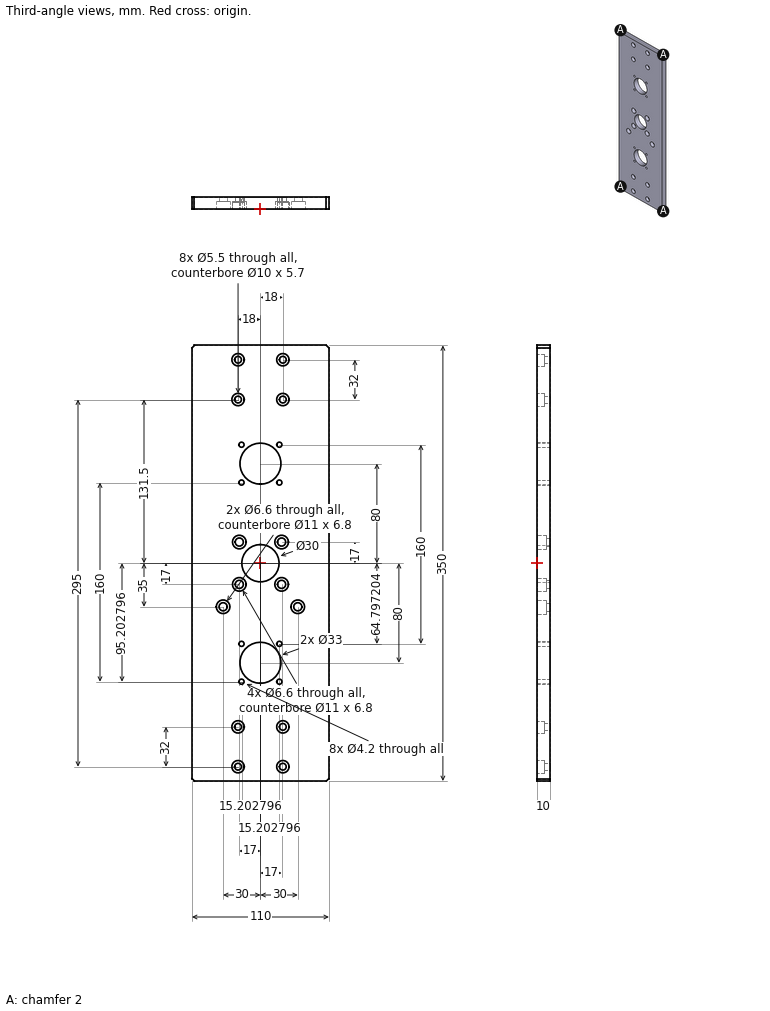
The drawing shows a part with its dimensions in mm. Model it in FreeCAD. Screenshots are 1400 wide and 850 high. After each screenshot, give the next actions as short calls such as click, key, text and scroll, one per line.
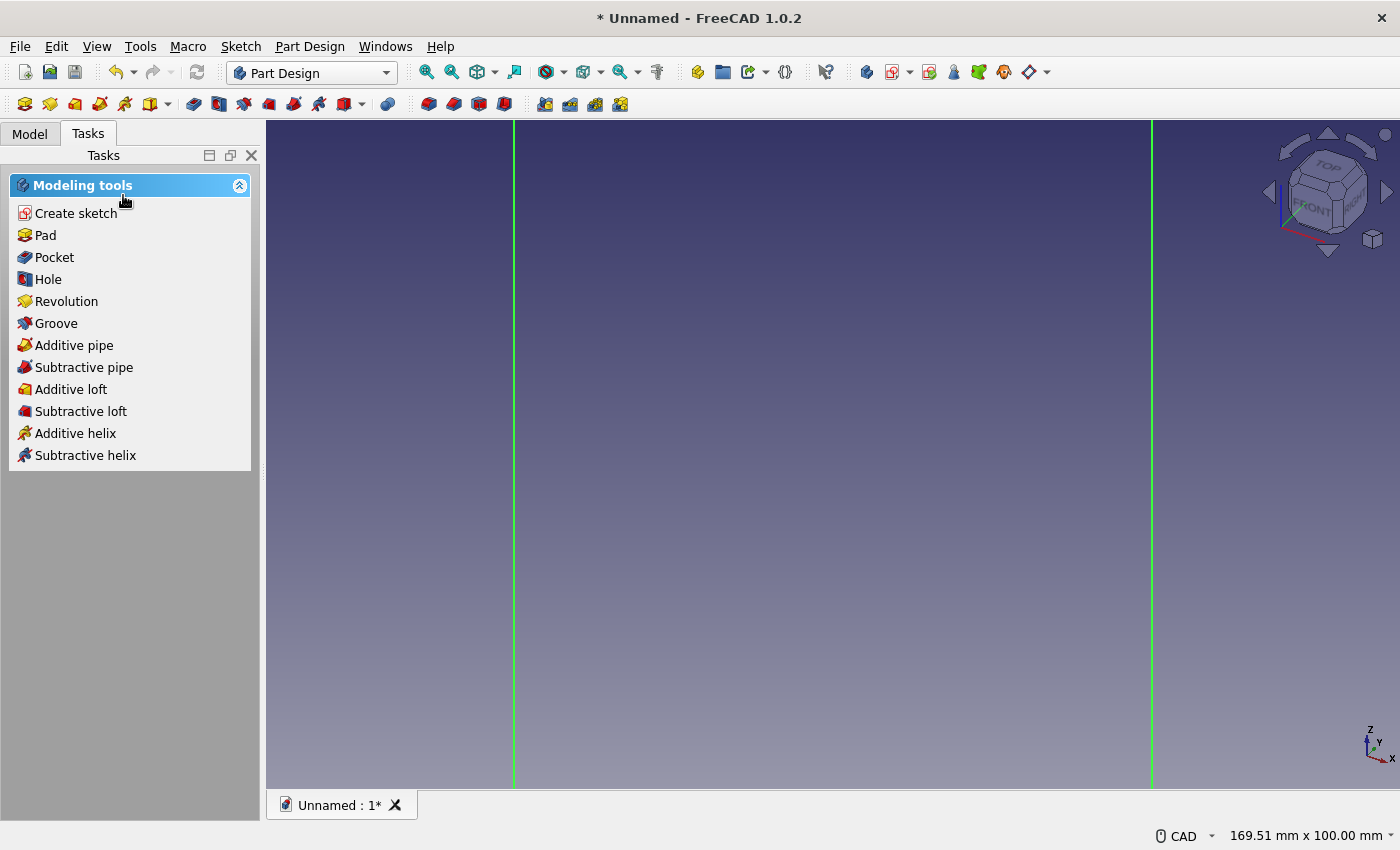
click(25, 104)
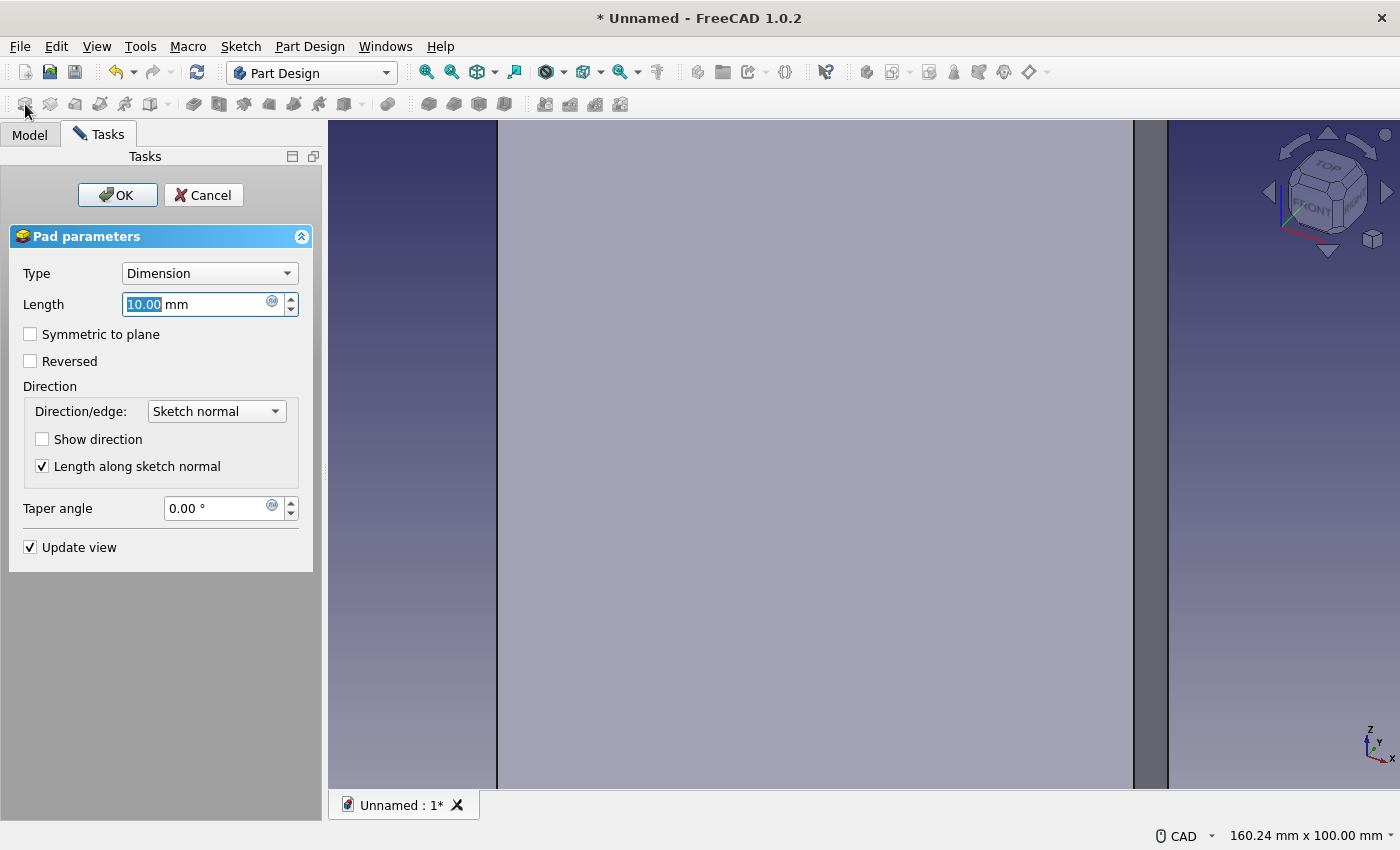
text(10)
key(Tab)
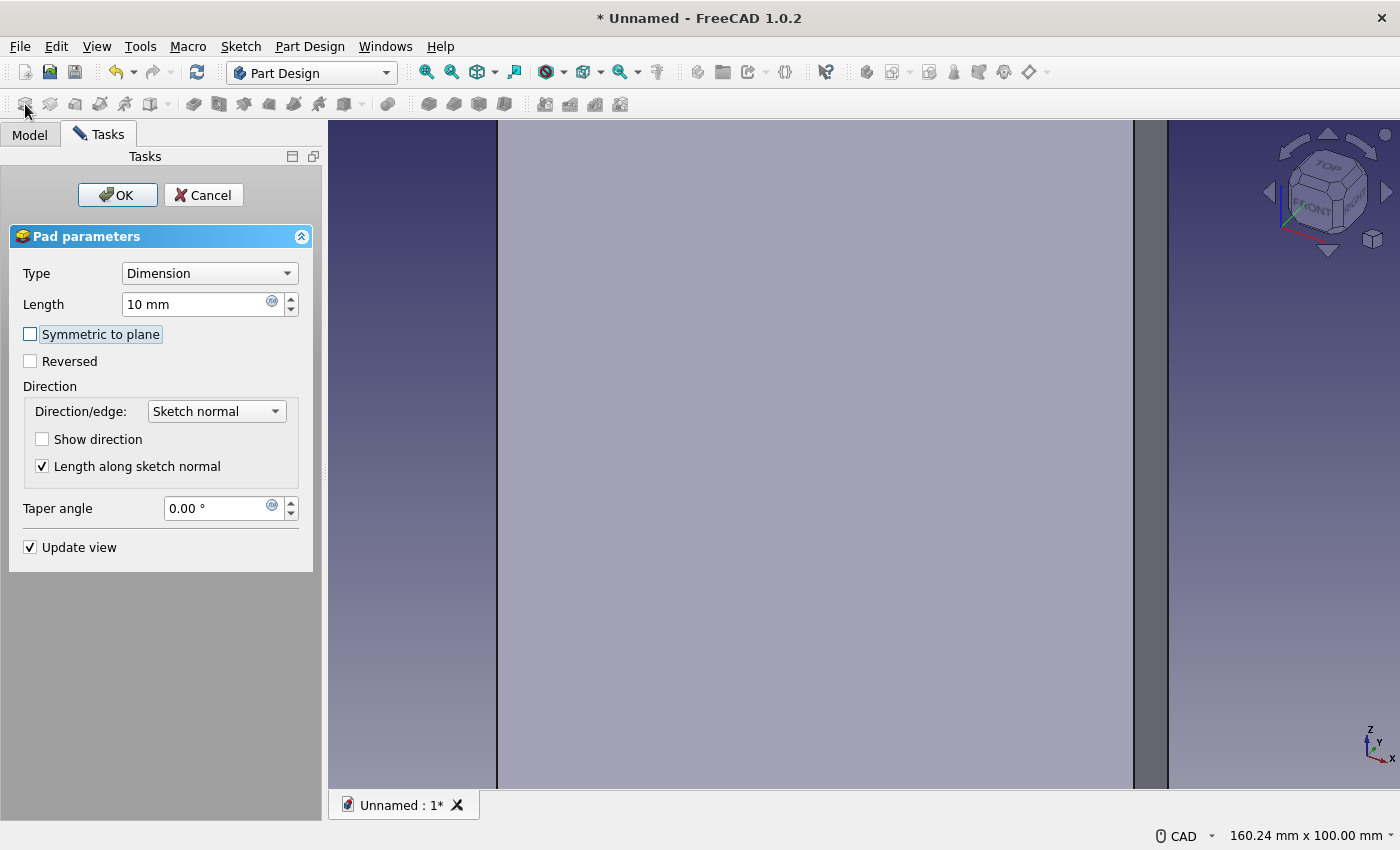
click(31, 361)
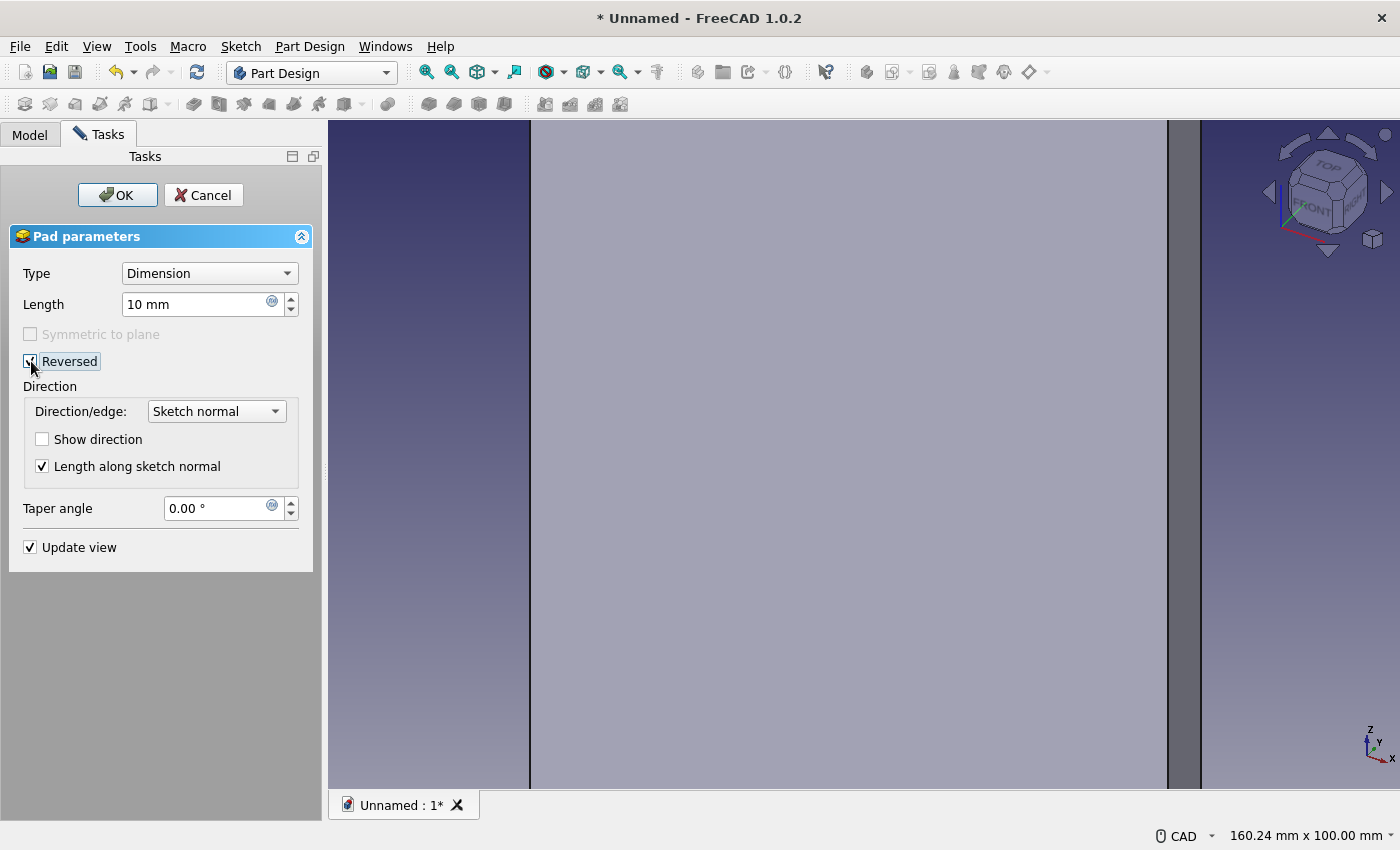
click(118, 195)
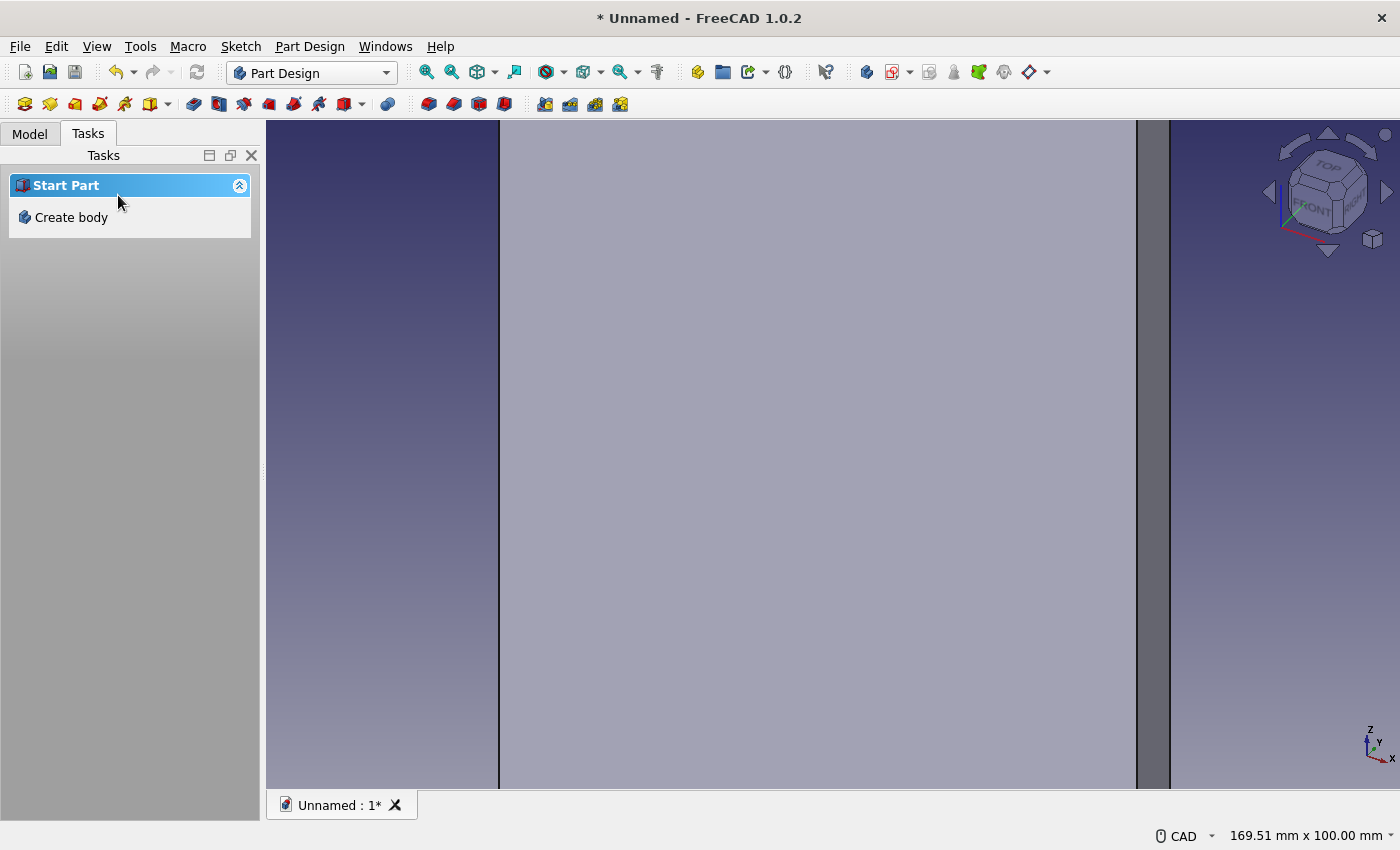
key(v)
key(f)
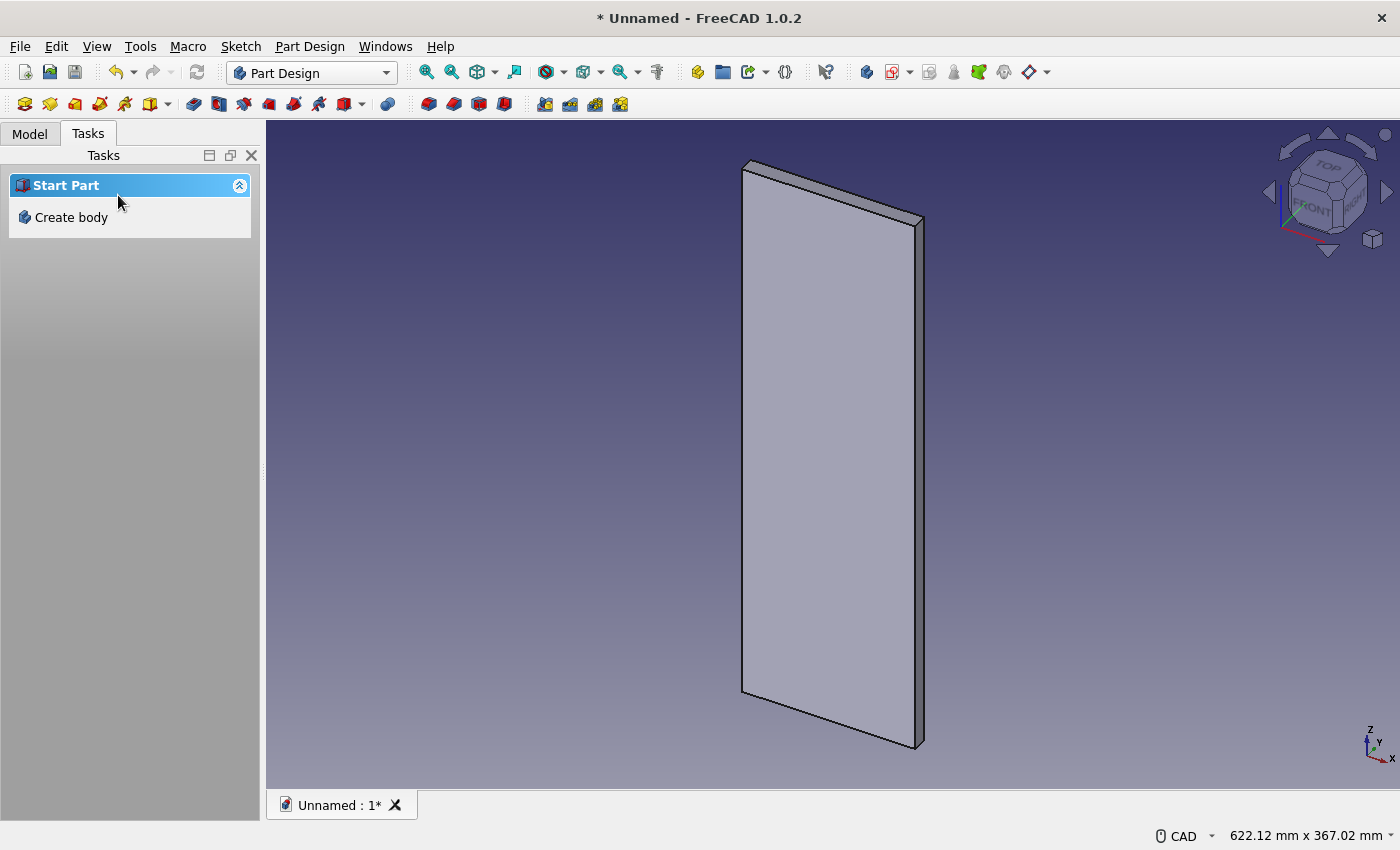
click(892, 72)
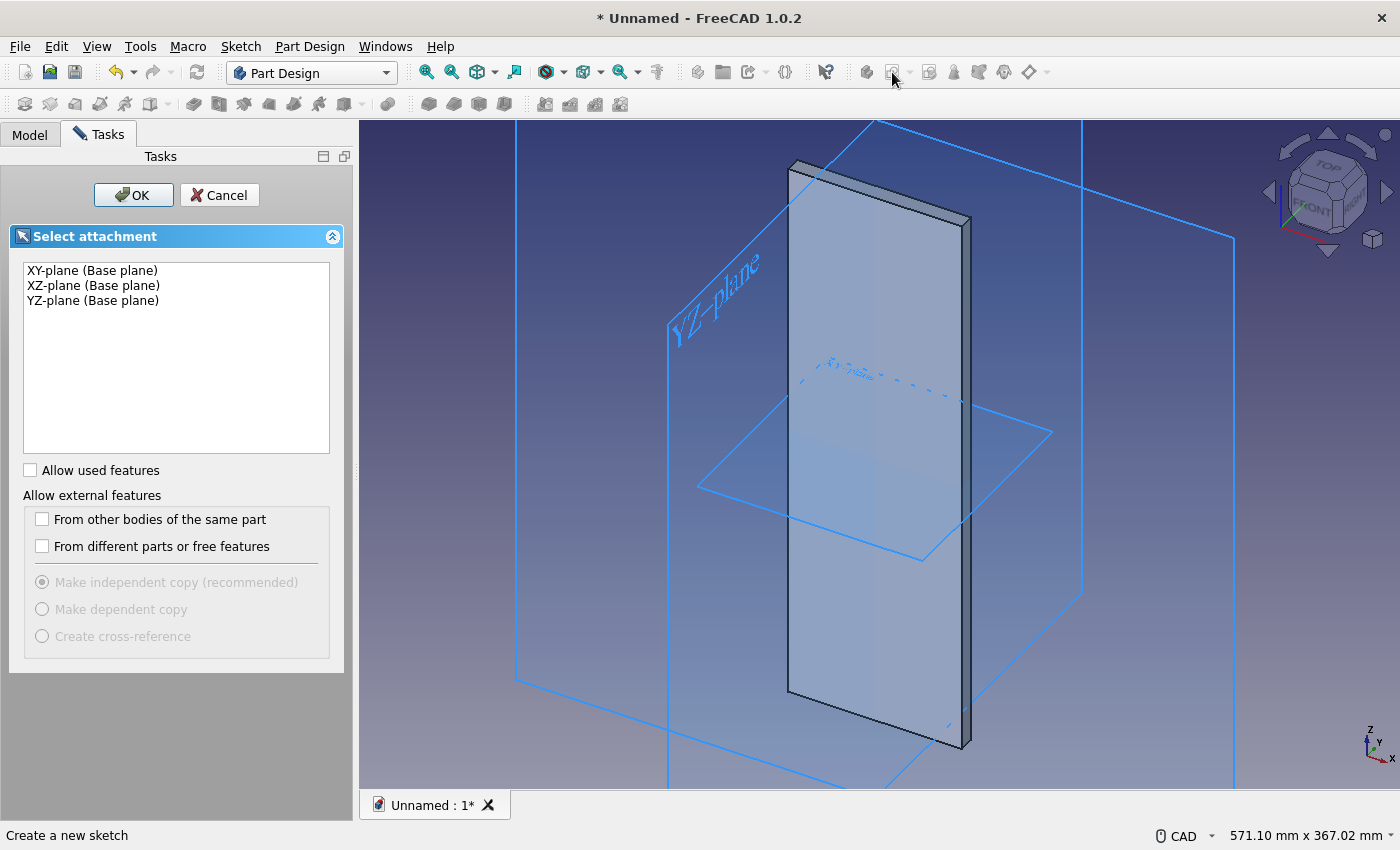
click(84, 286)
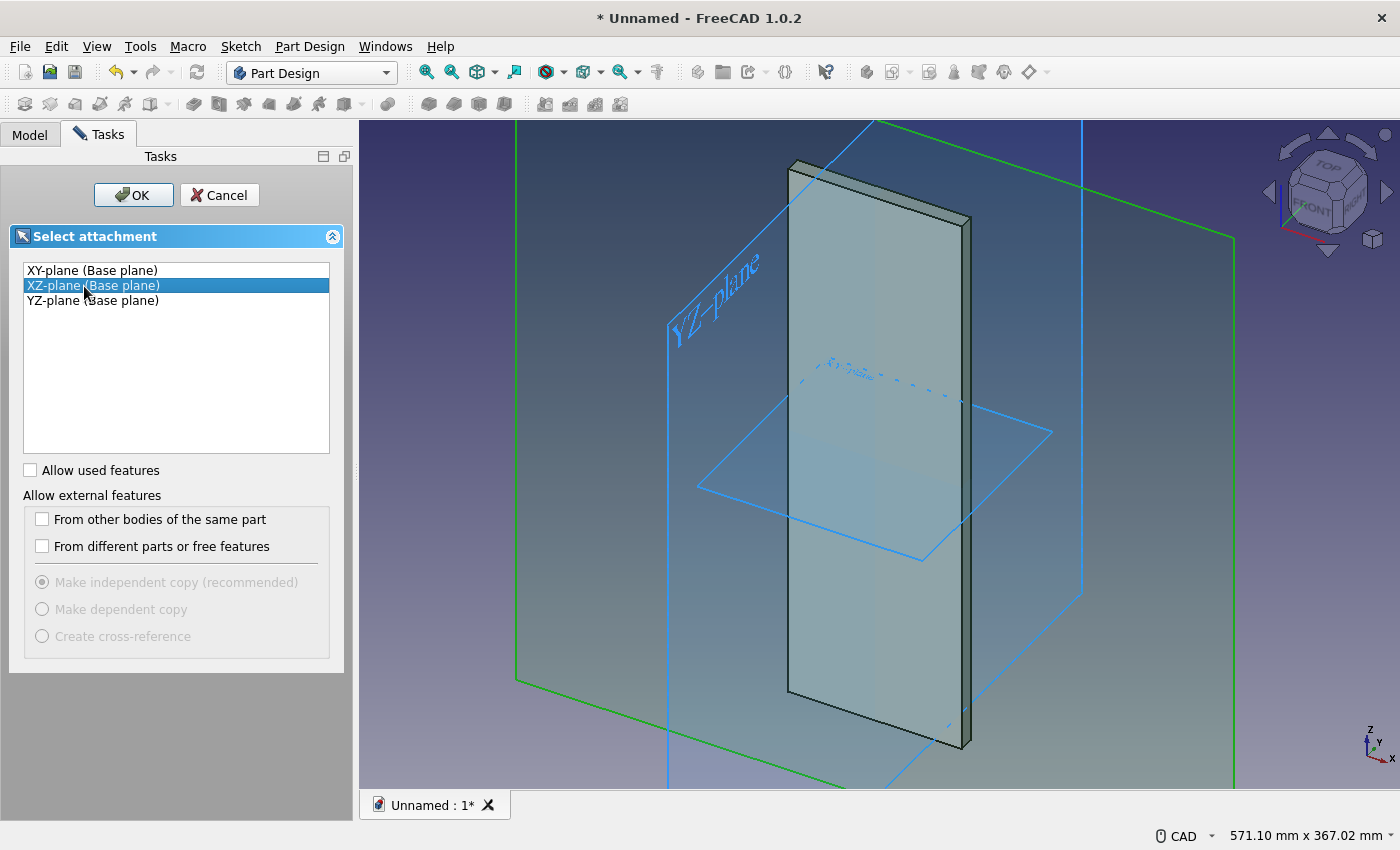
click(134, 195)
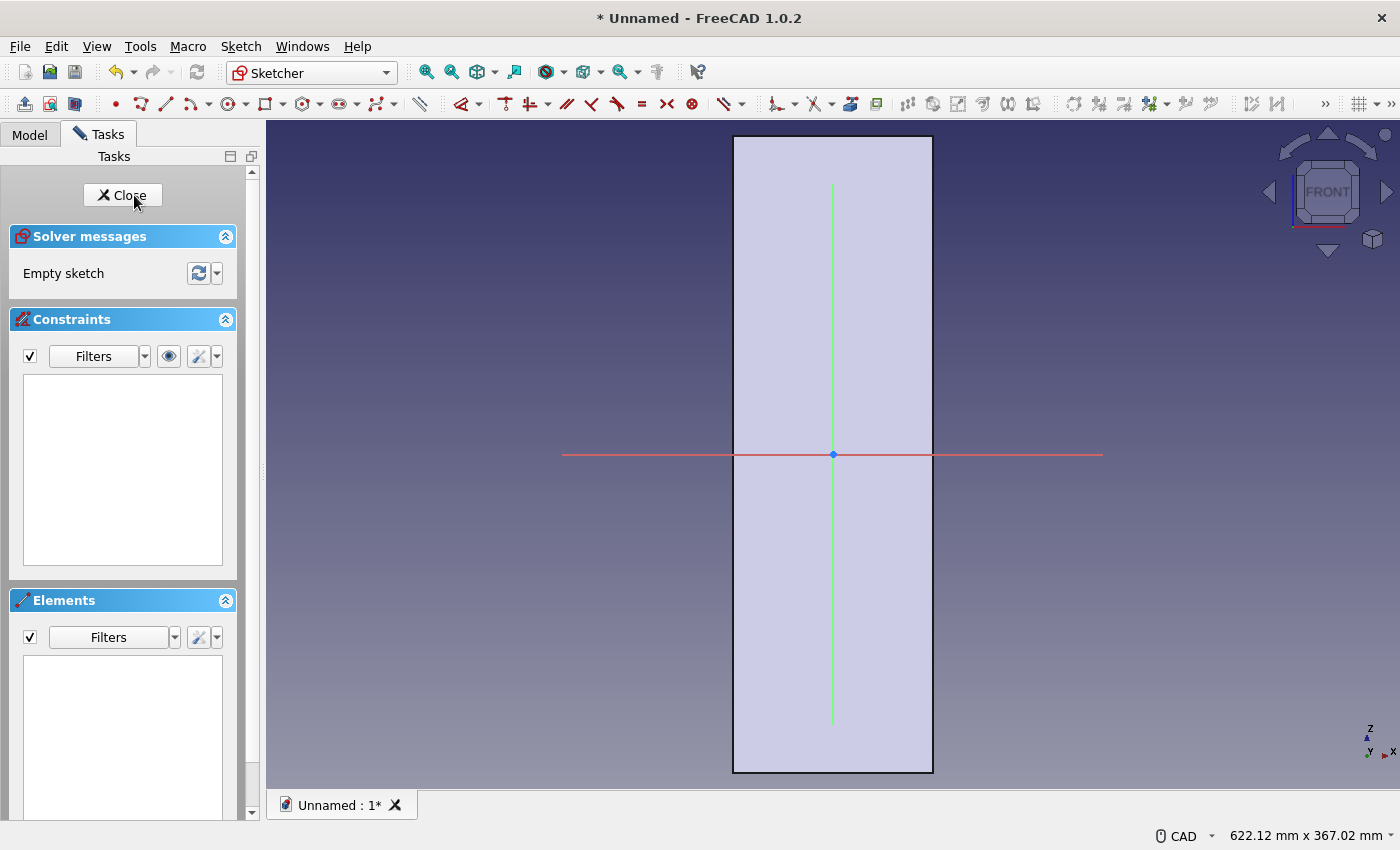
scroll(625, 454, down, 2)